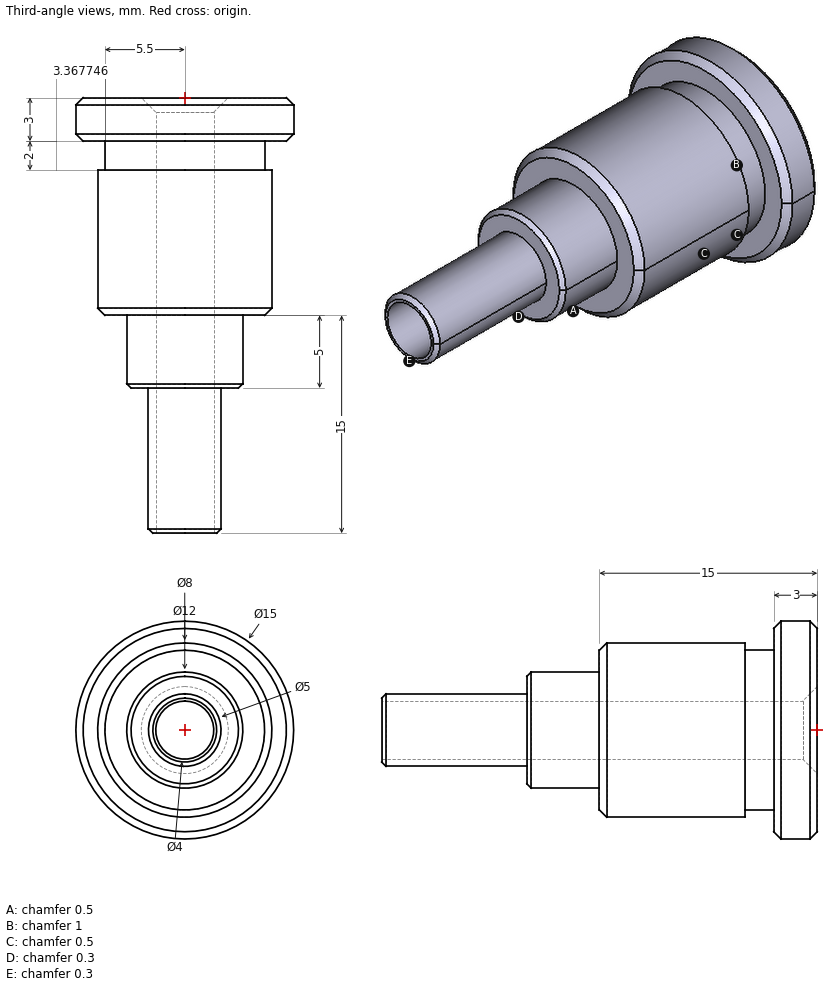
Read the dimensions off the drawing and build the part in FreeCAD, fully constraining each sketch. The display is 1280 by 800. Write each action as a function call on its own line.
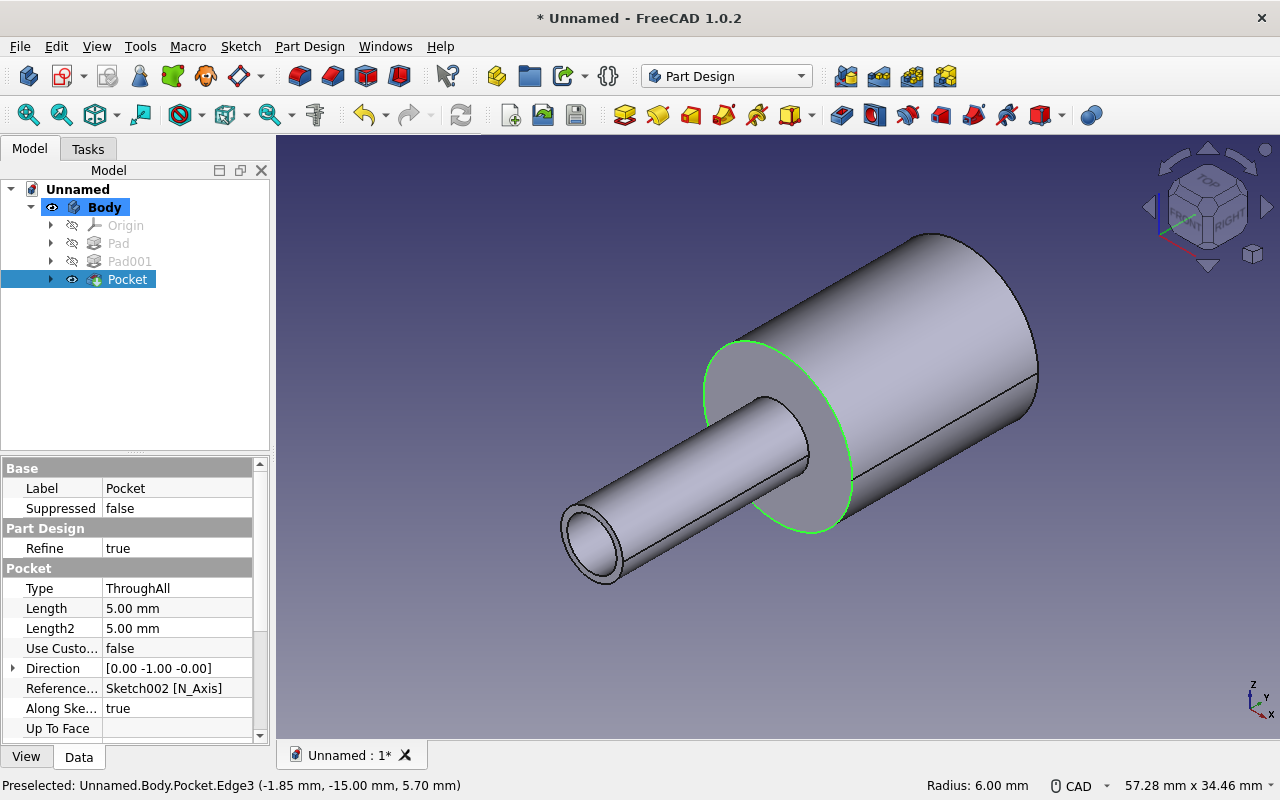
click(333, 76)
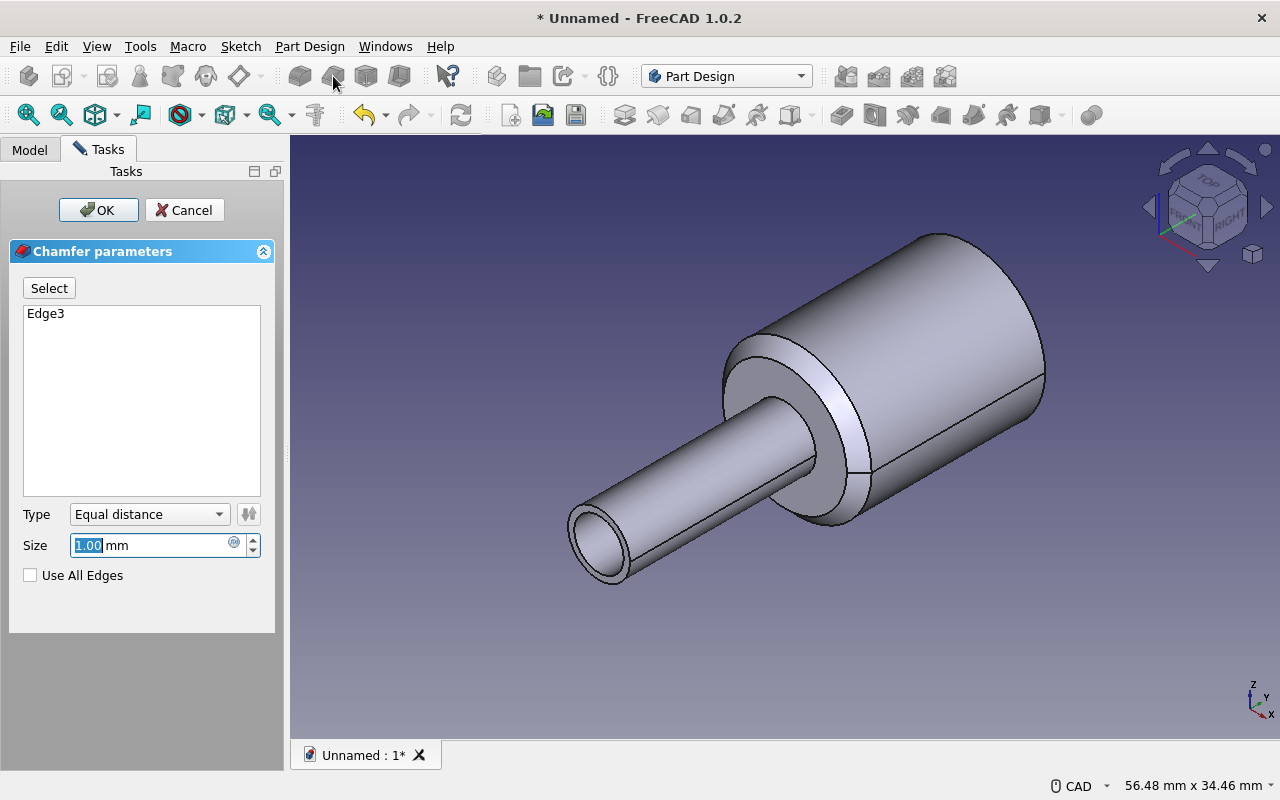
text(0.5)
key(Tab)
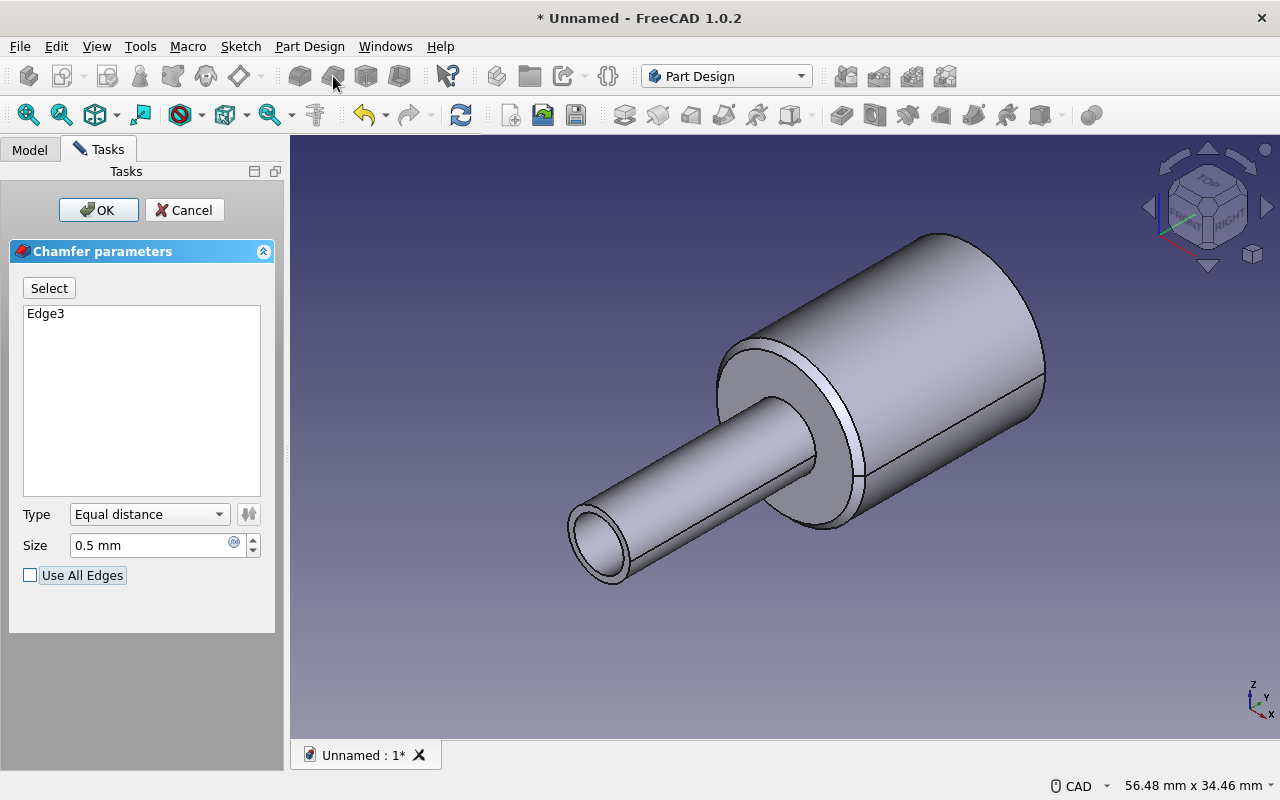
click(99, 210)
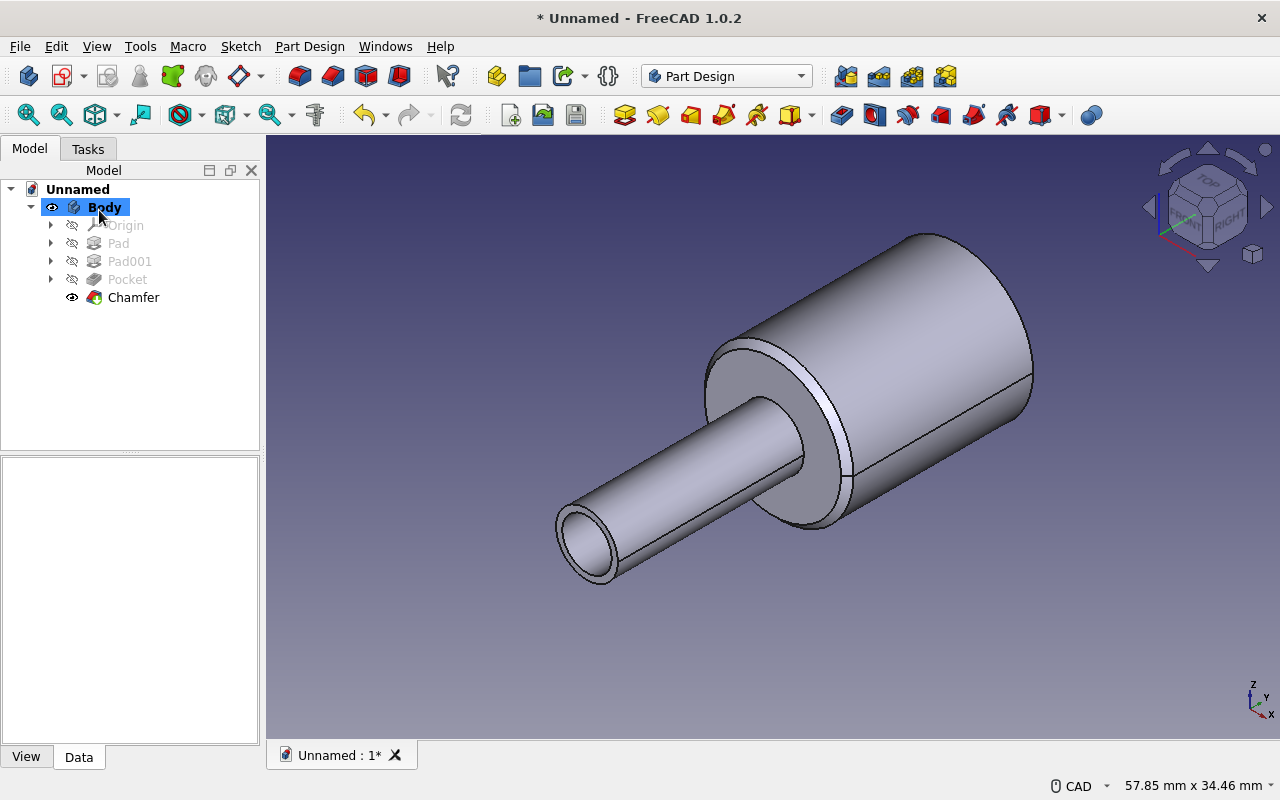
click(62, 76)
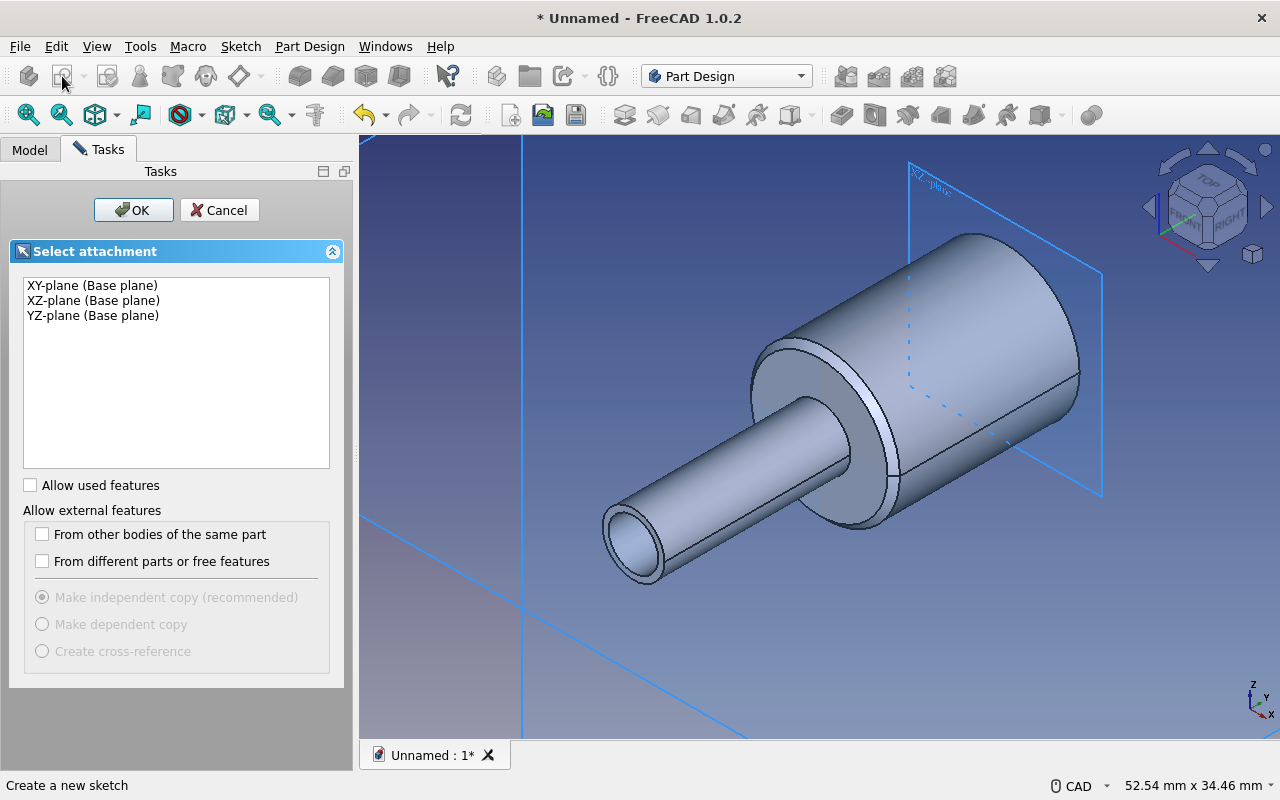
click(84, 300)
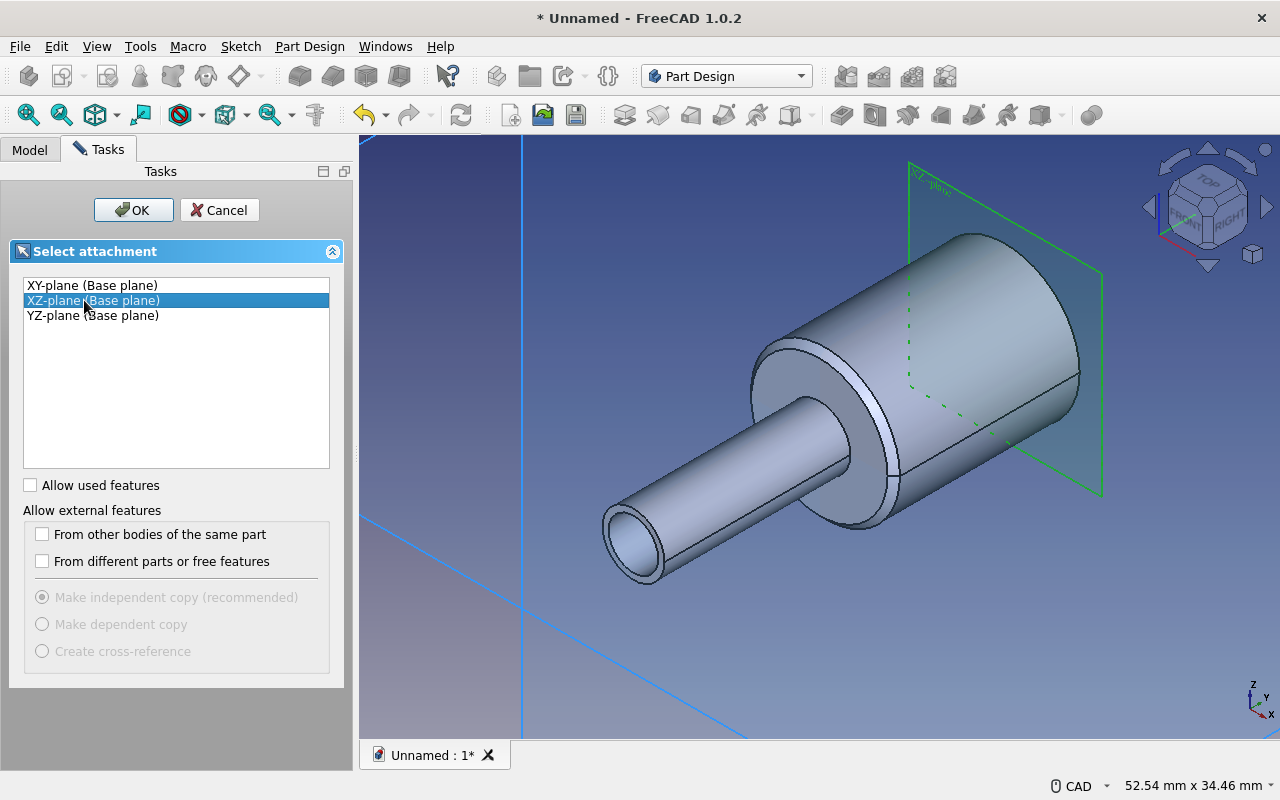
click(134, 210)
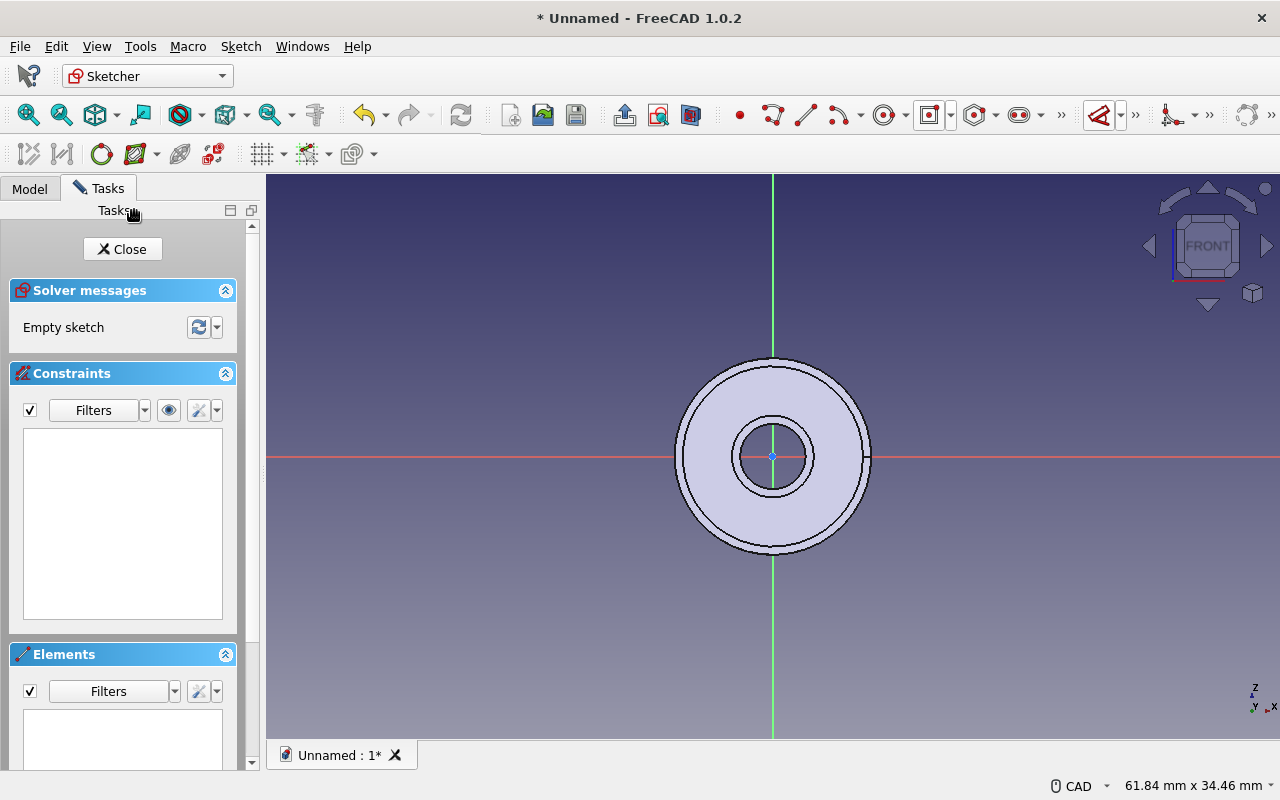
click(691, 116)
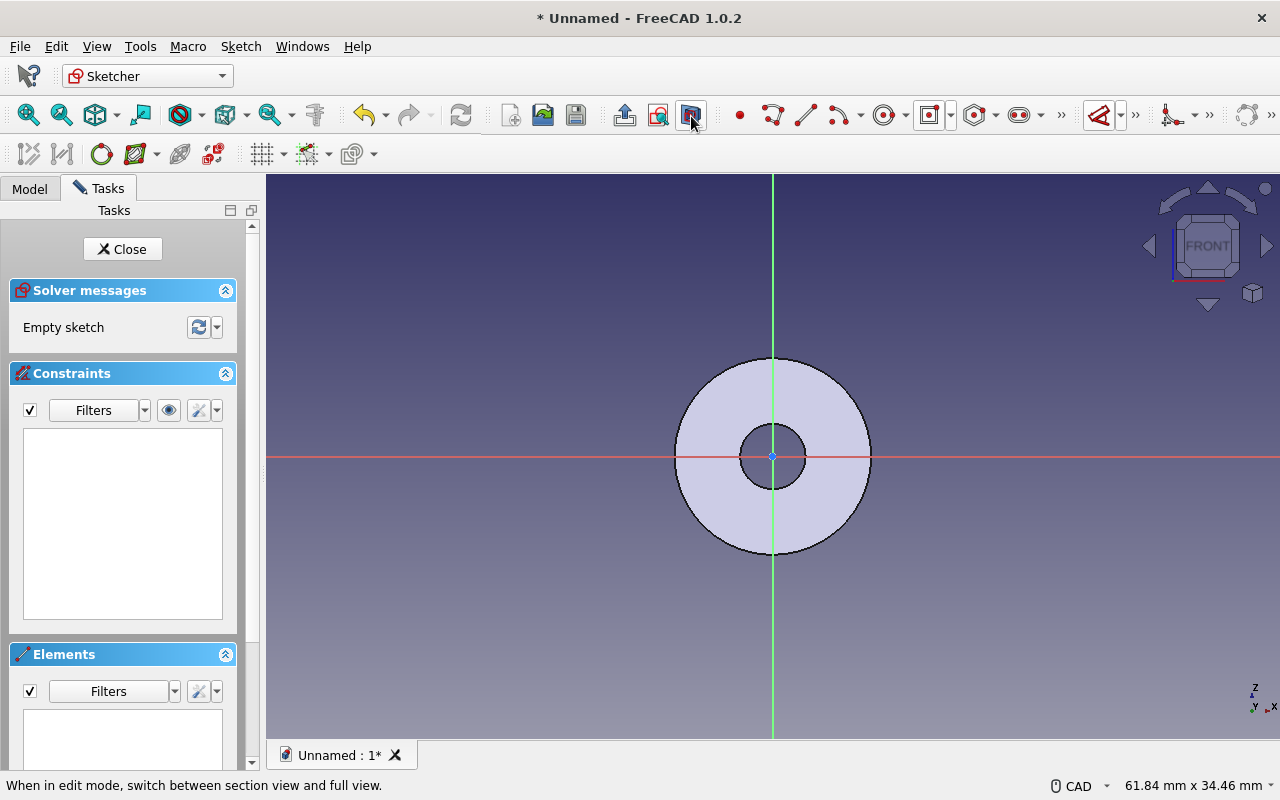
scroll(912, 456, up, 2)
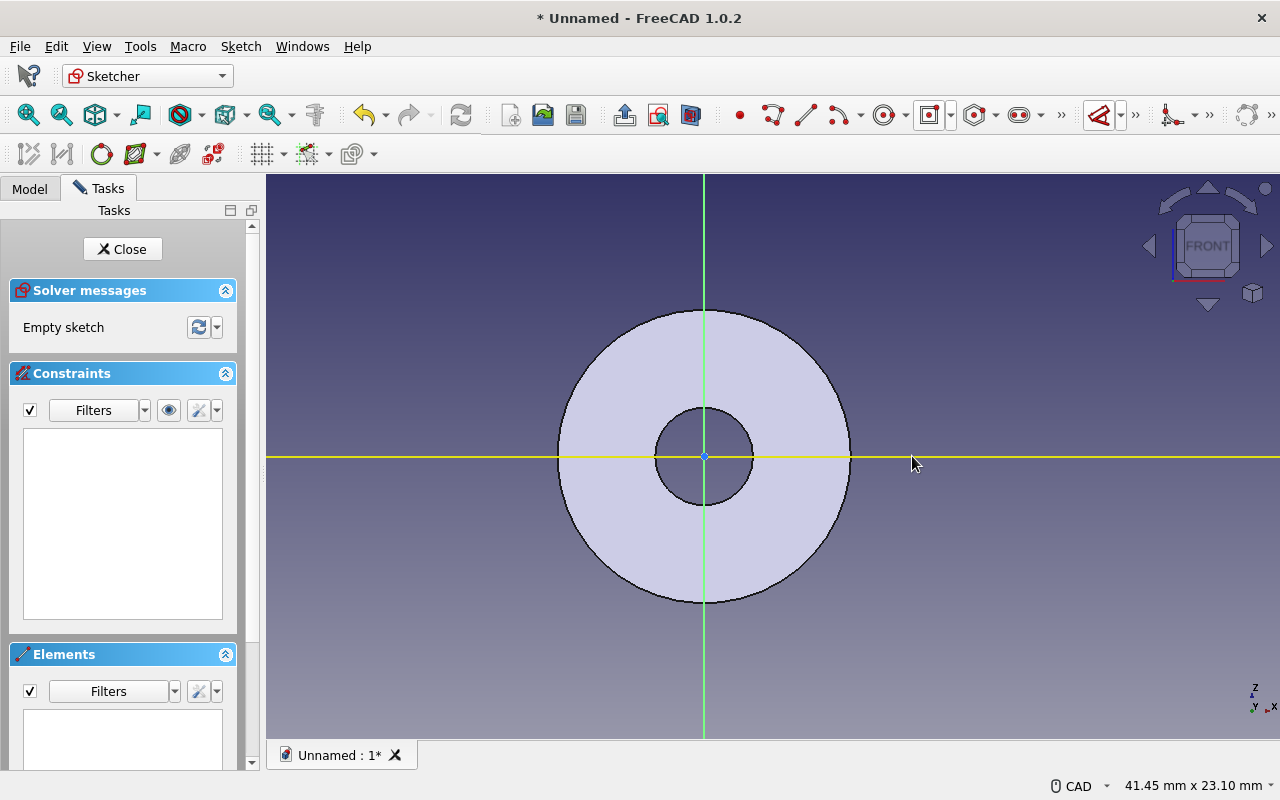
click(884, 116)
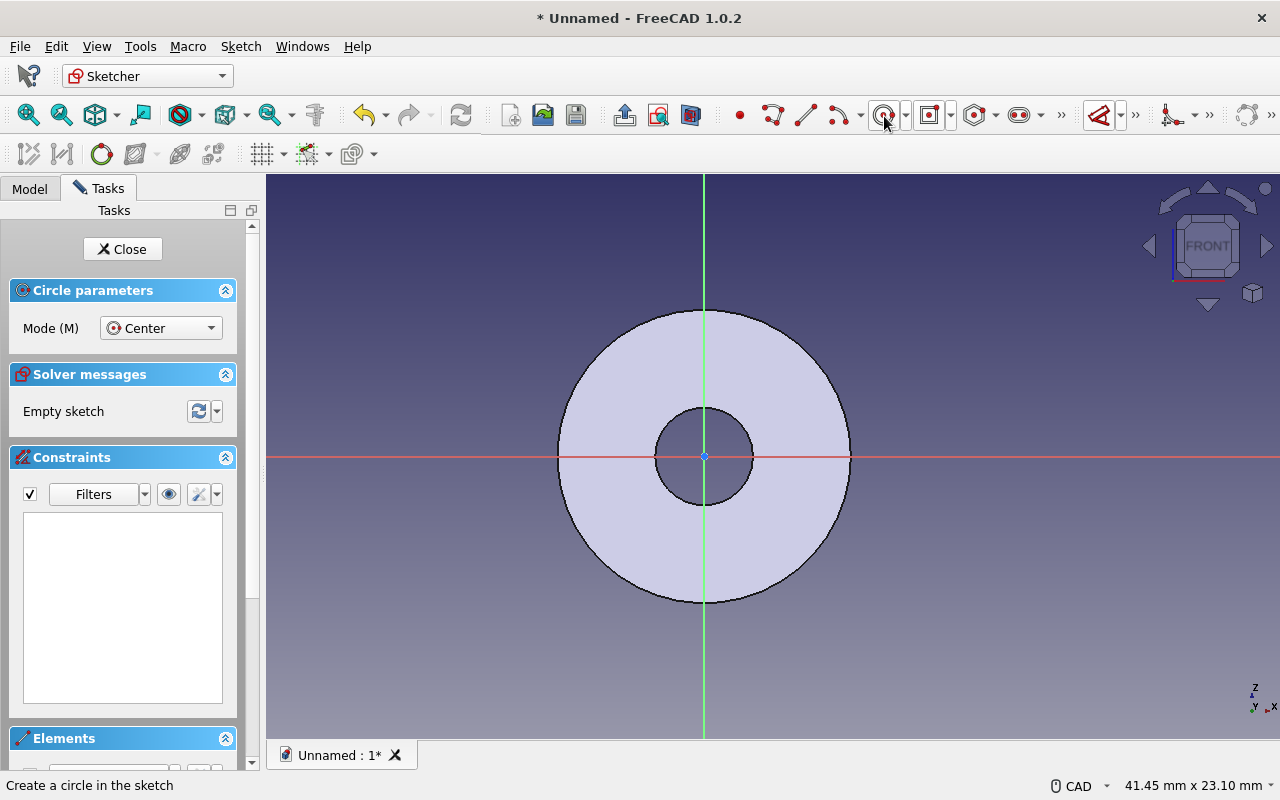
click(704, 456)
move(834, 327)